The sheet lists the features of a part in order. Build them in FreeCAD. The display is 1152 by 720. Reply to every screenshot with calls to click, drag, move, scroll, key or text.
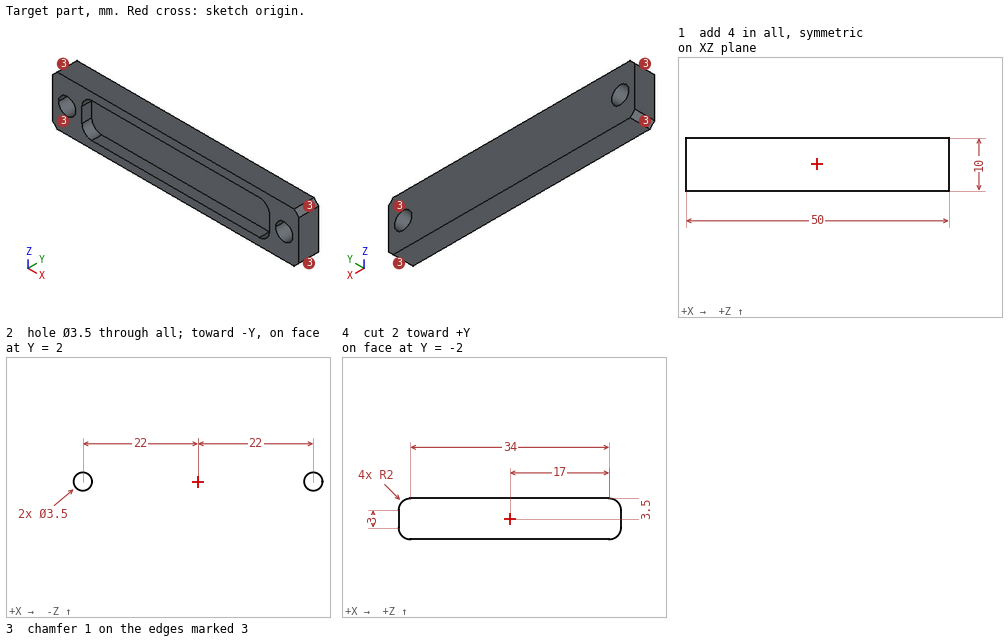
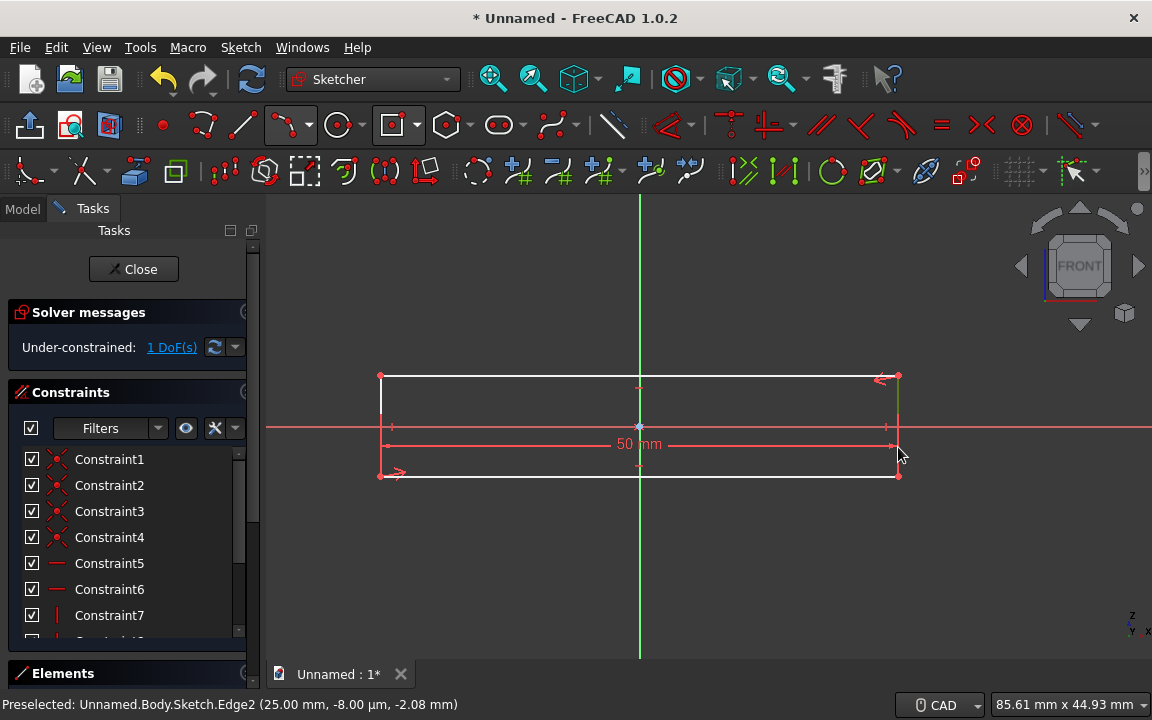
key(i)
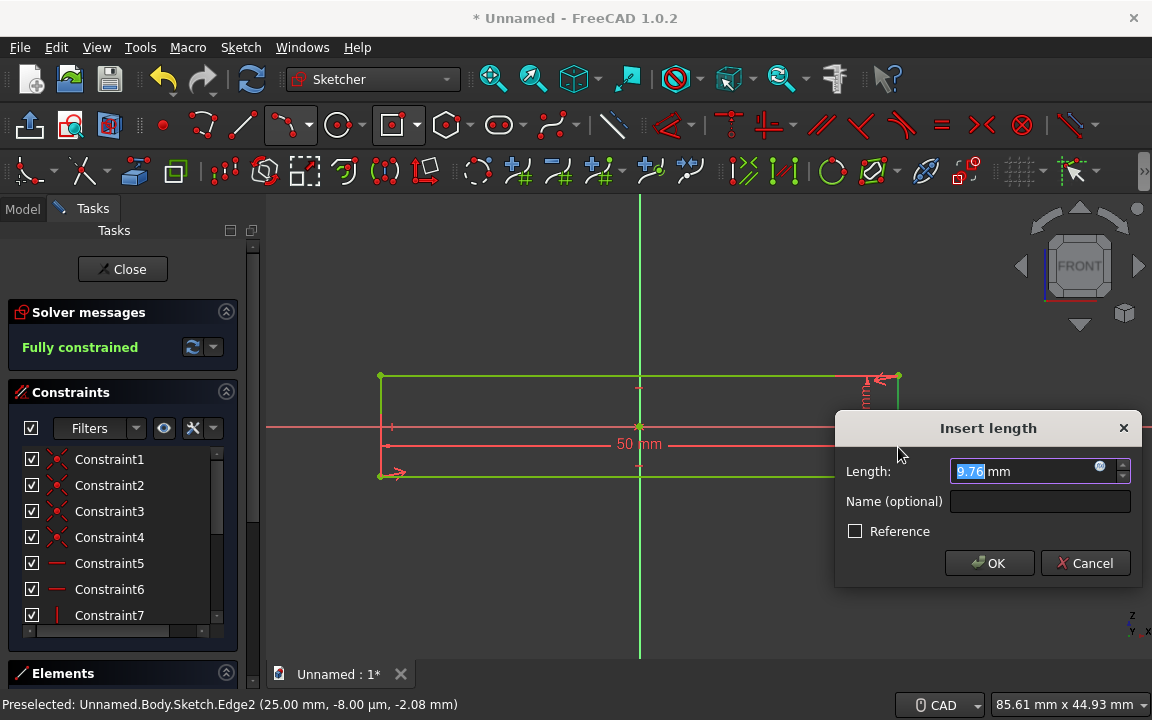
text(10)
key(Return)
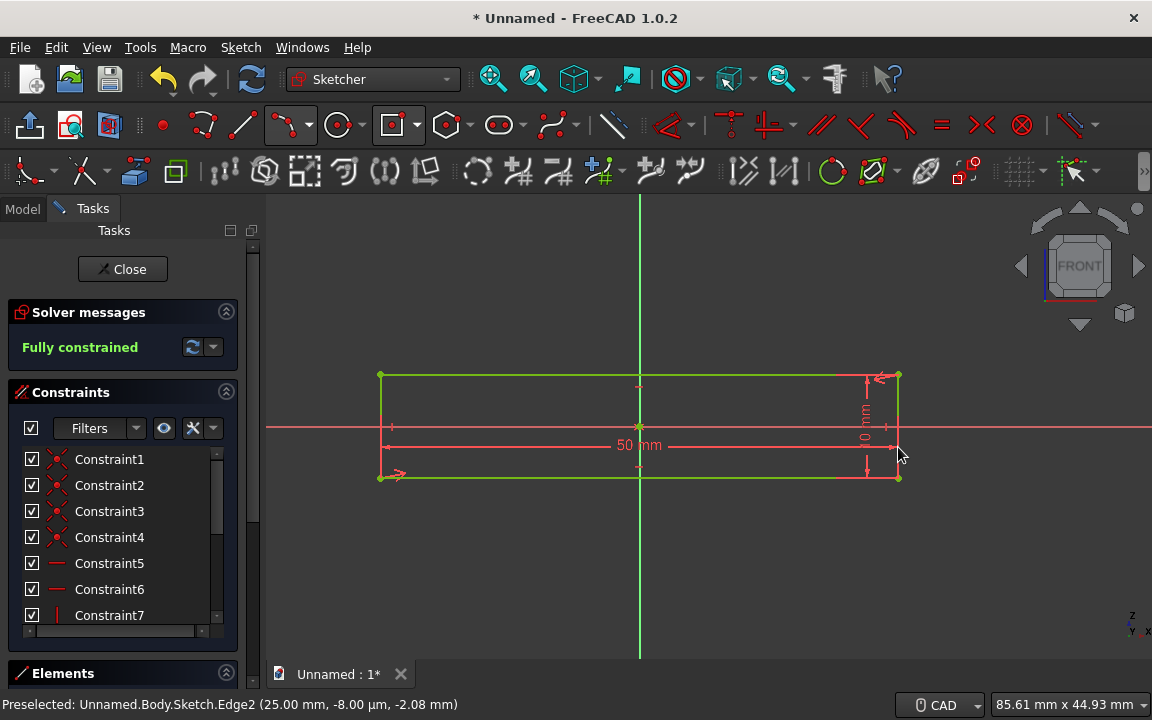
click(123, 269)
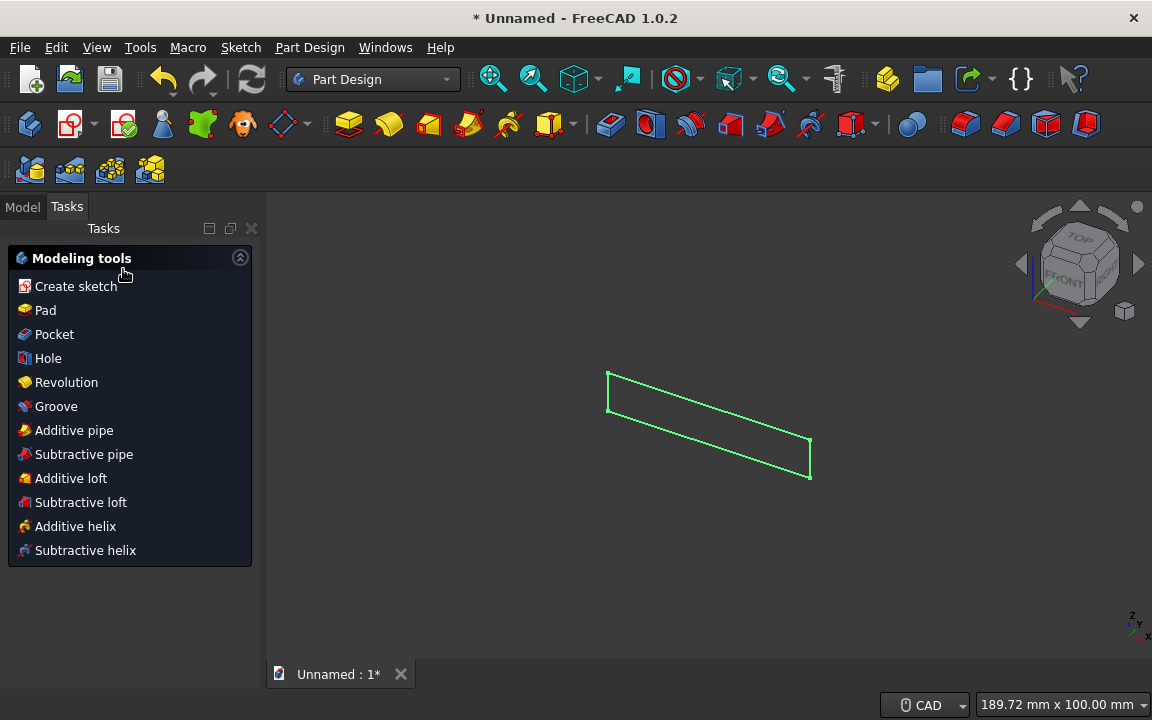
click(350, 124)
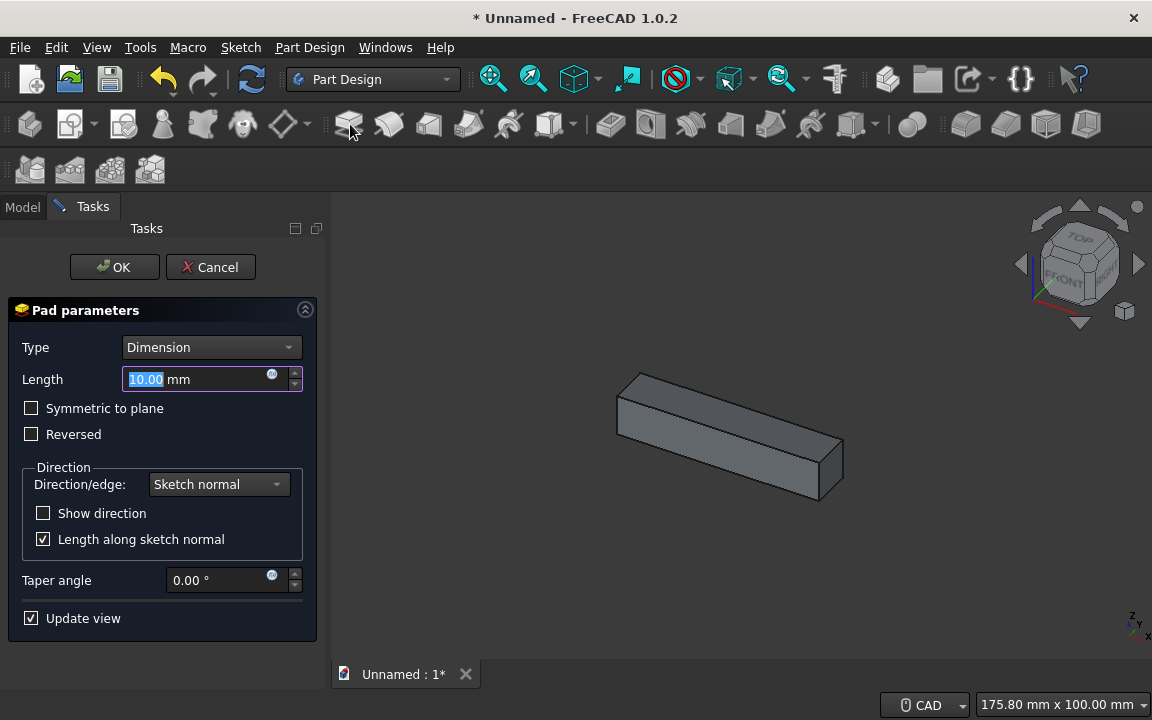
text(4)
key(Tab)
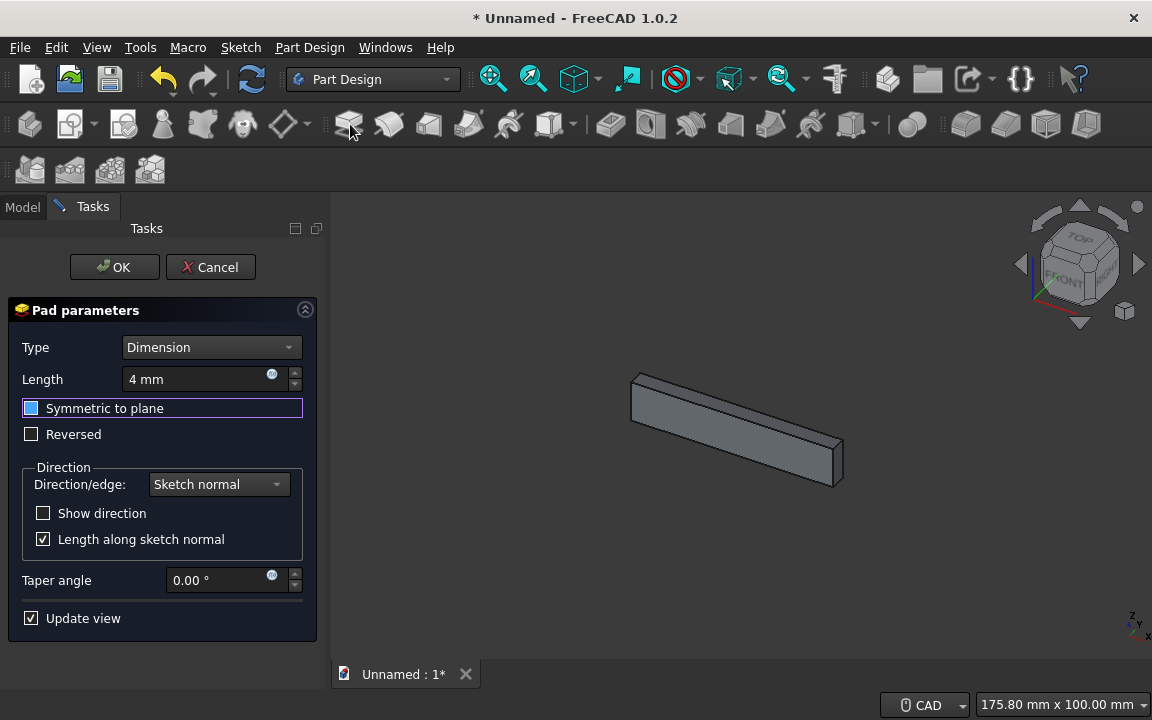
click(30, 408)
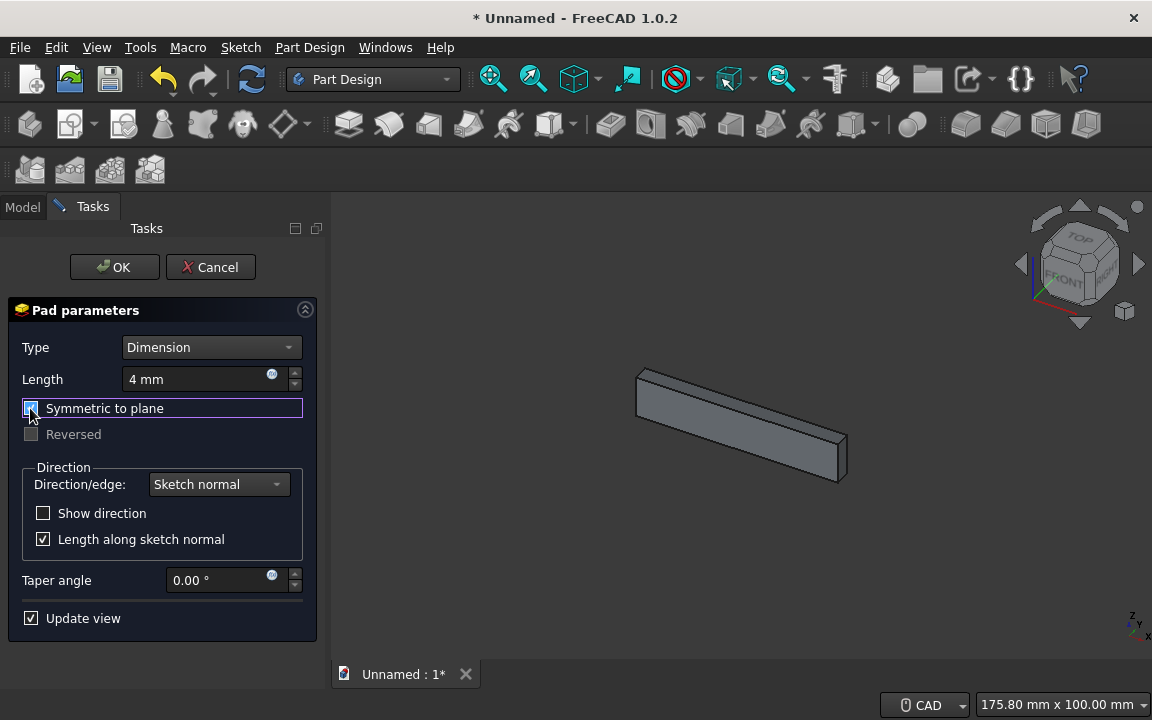
click(115, 267)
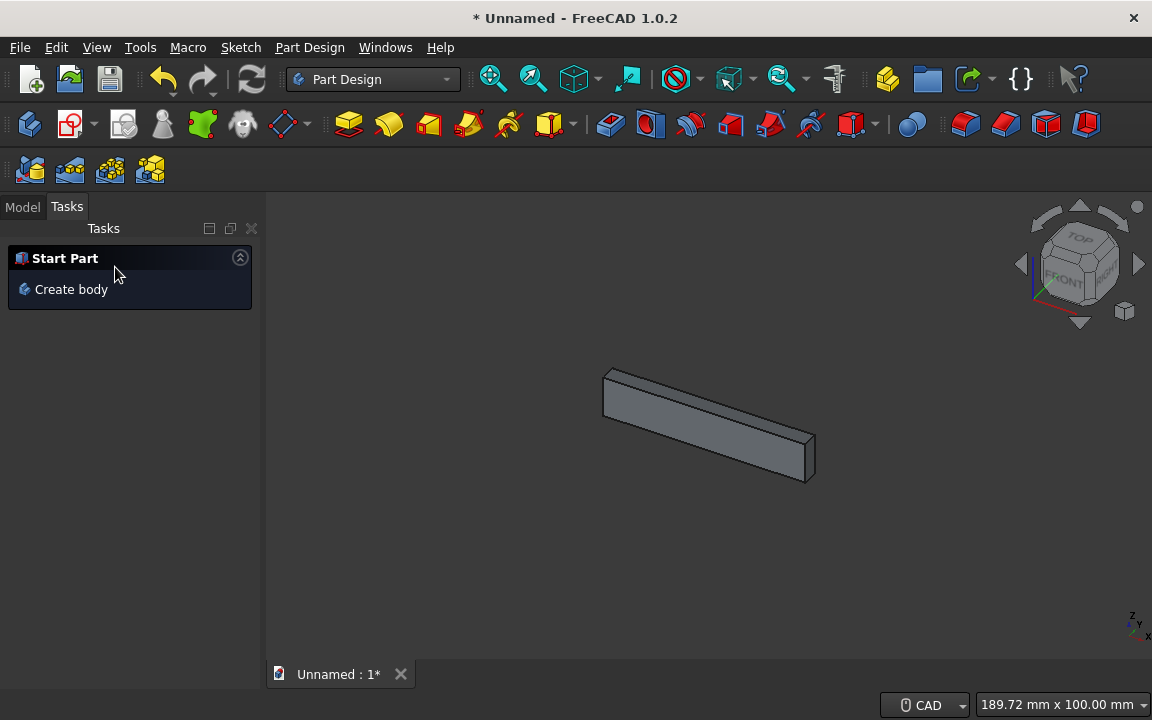
click(494, 80)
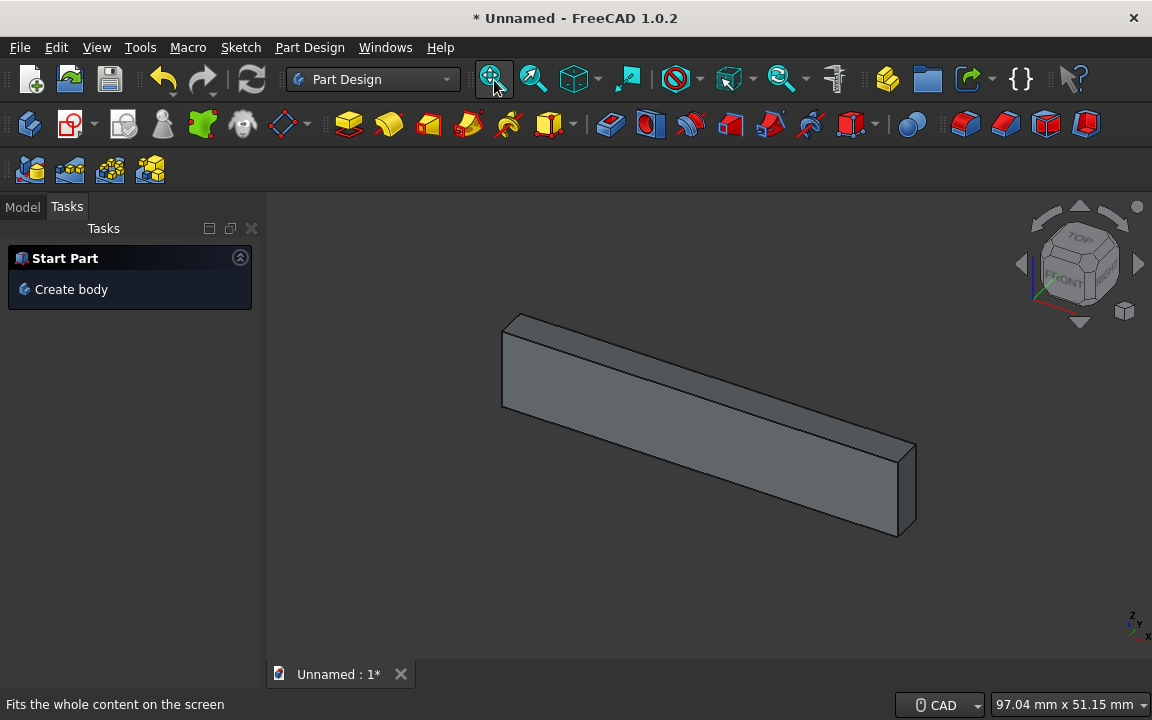
key(4)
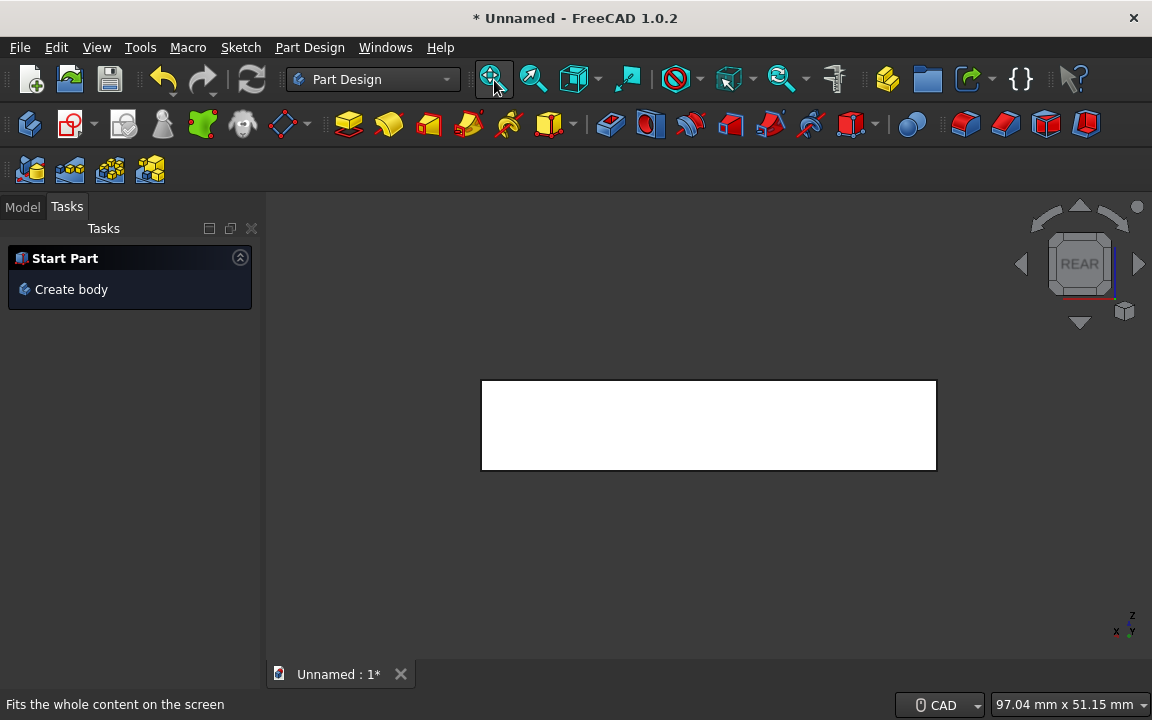
click(579, 424)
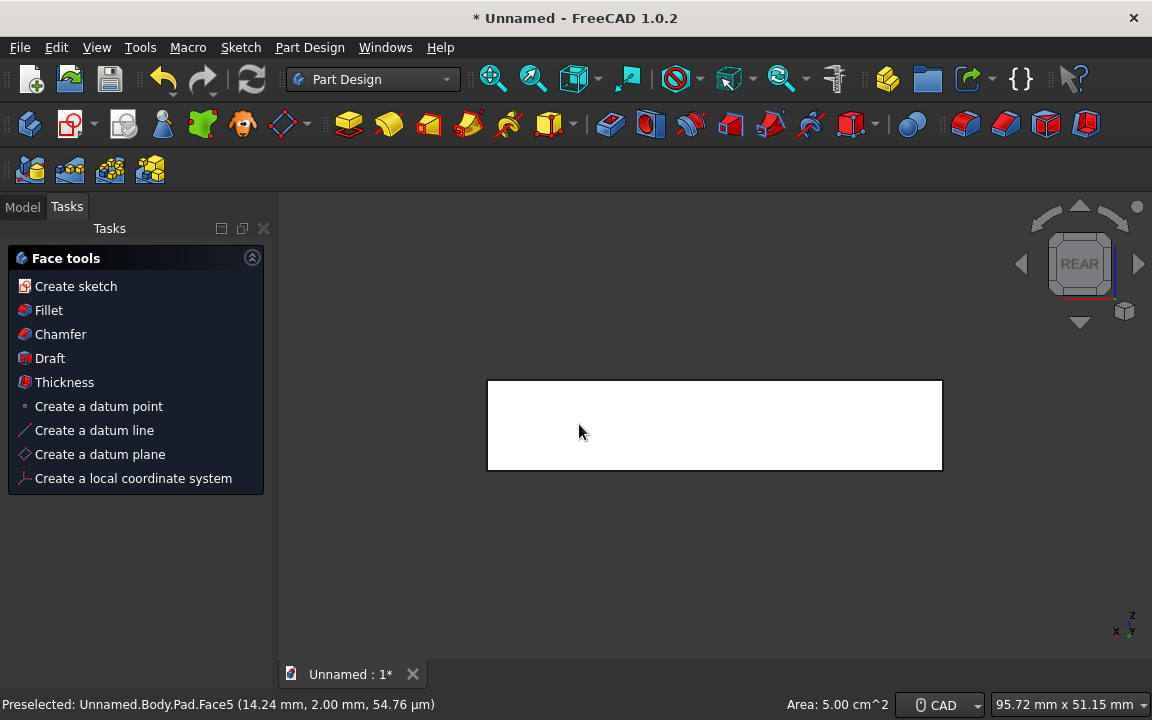
click(70, 124)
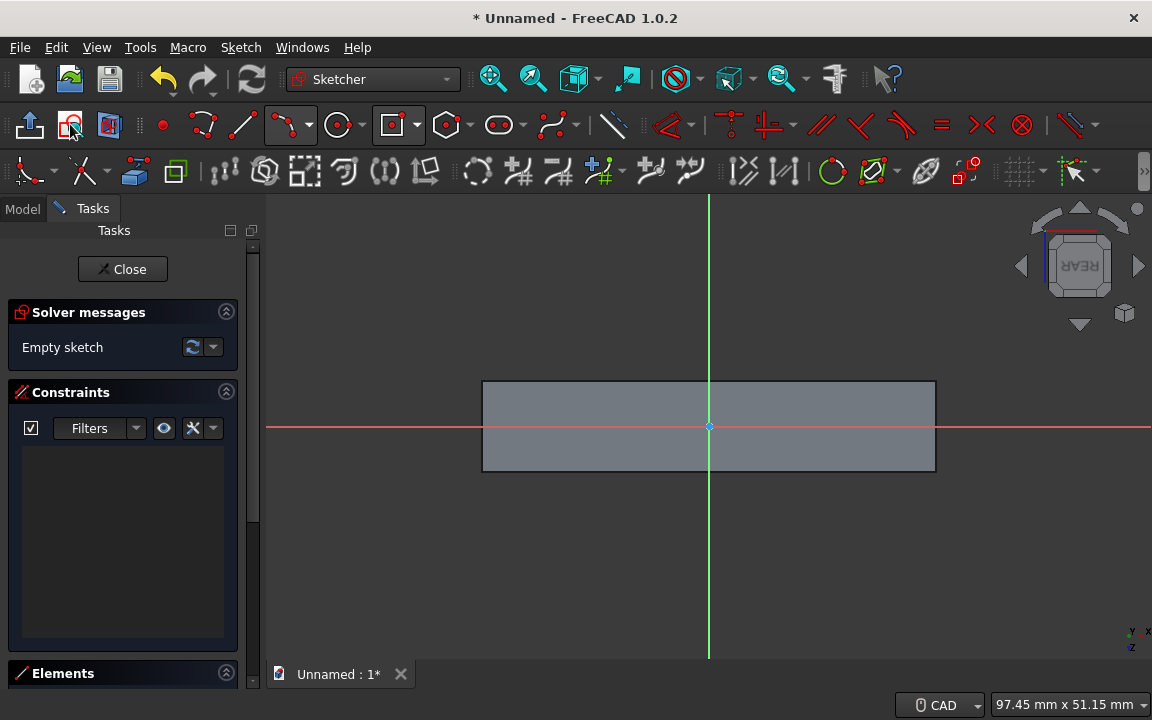
click(338, 126)